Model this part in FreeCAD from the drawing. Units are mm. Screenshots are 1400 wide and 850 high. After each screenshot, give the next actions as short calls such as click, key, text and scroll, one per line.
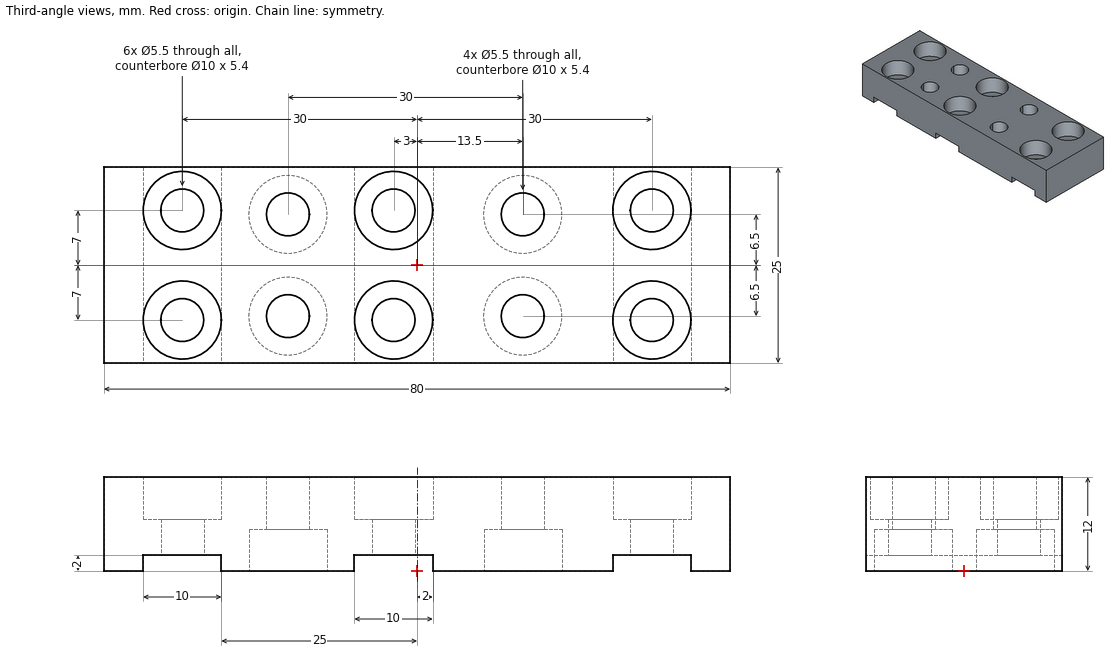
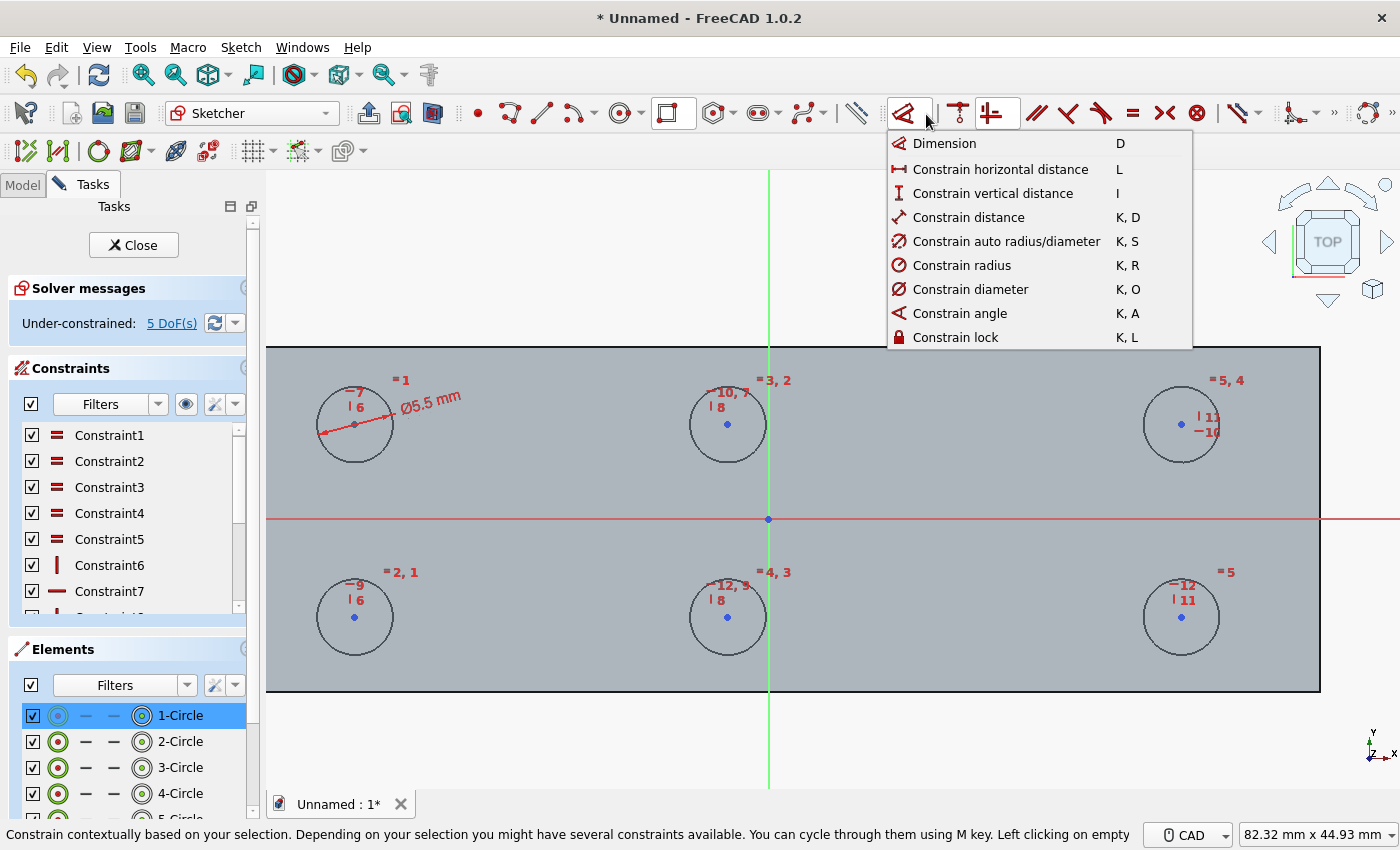
click(1040, 193)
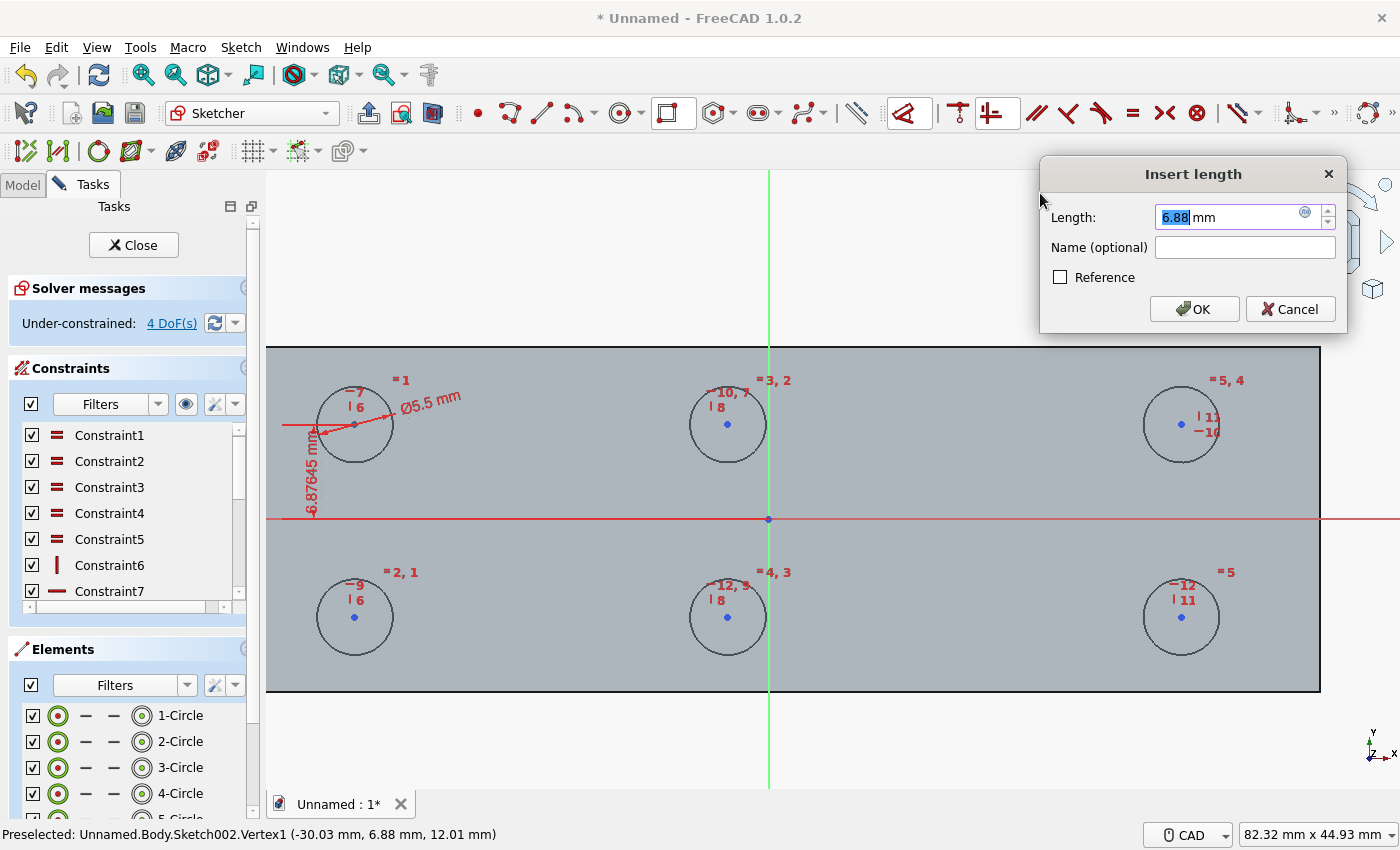
text(7)
key(Return)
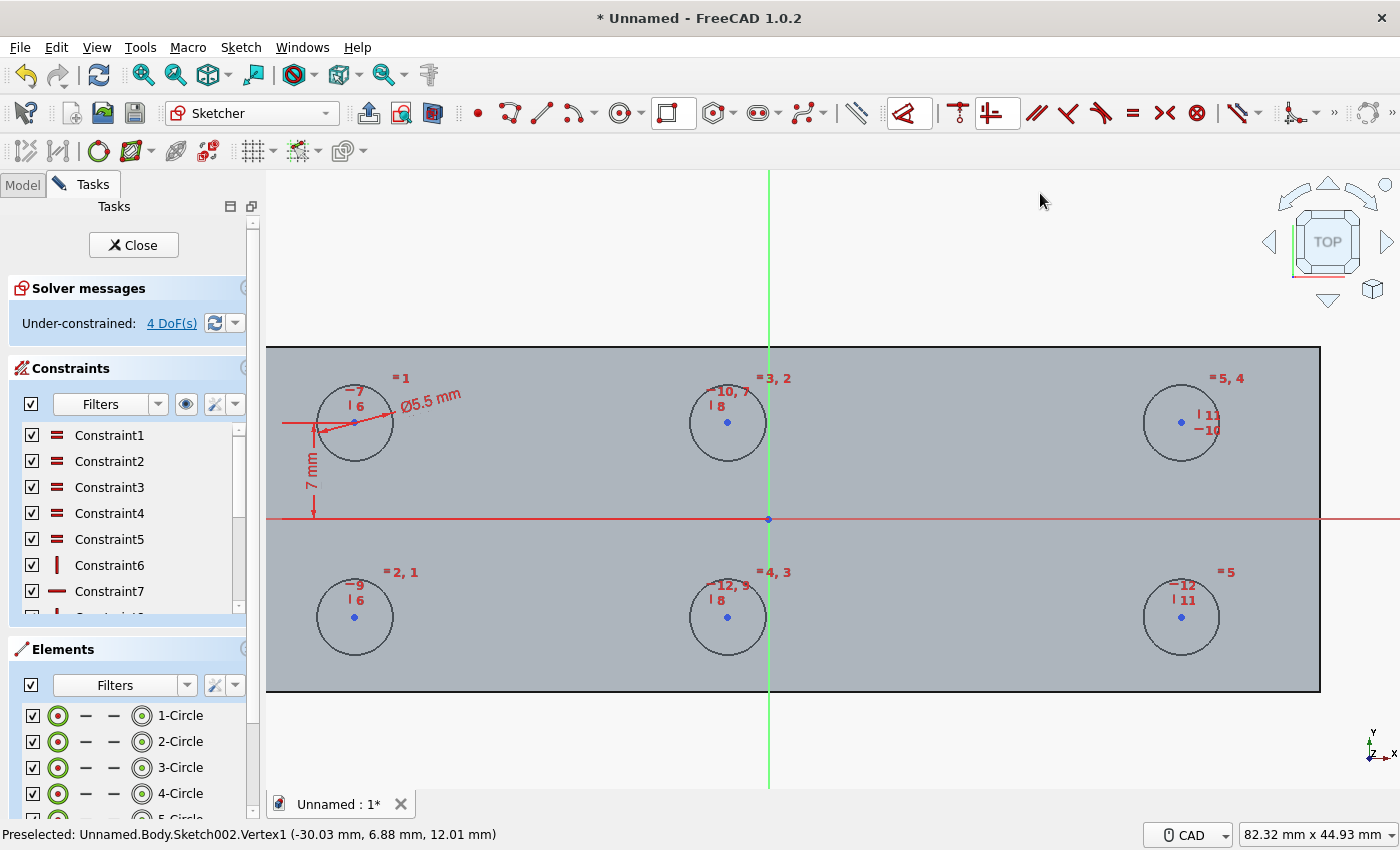
click(355, 617)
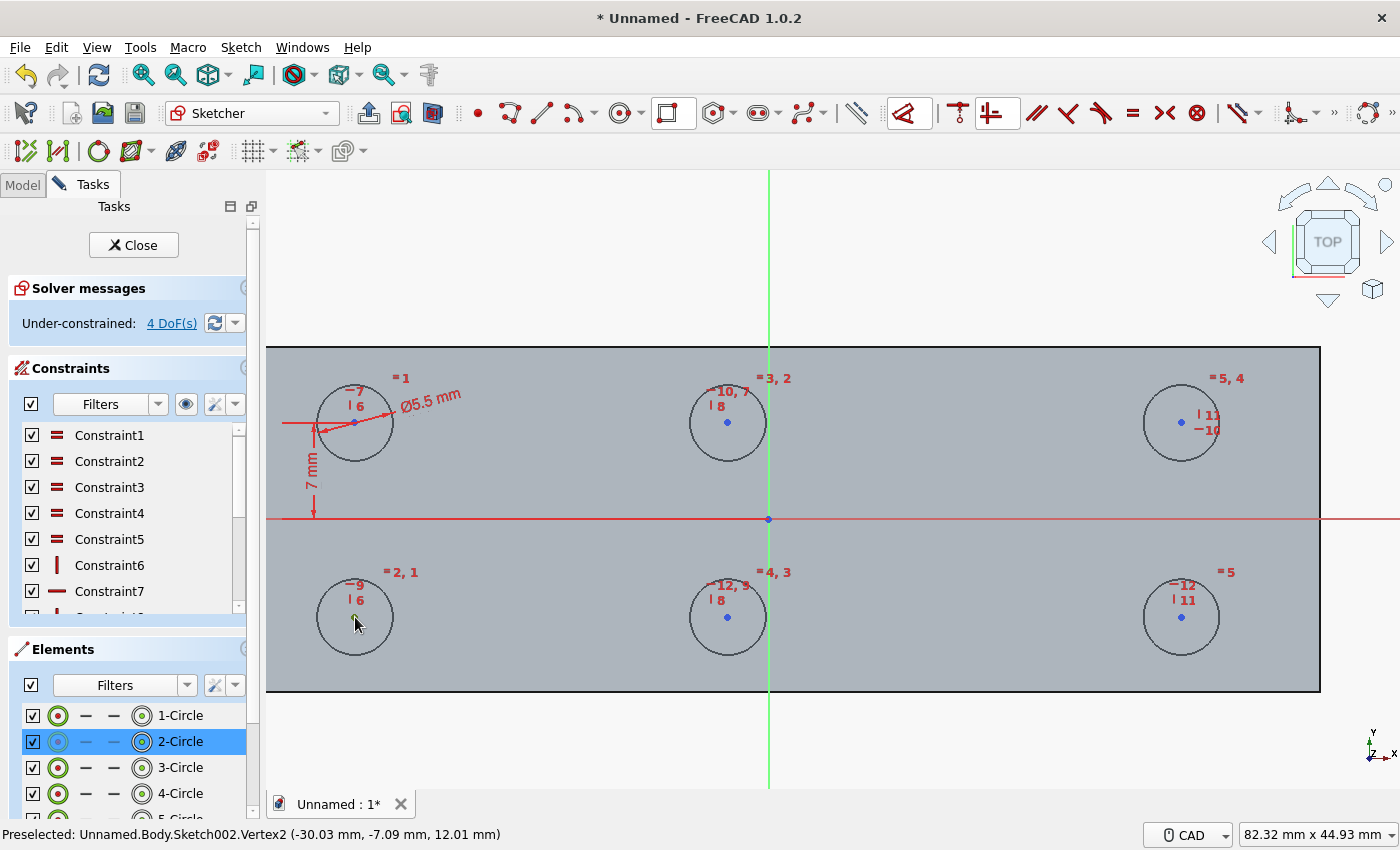
click(926, 114)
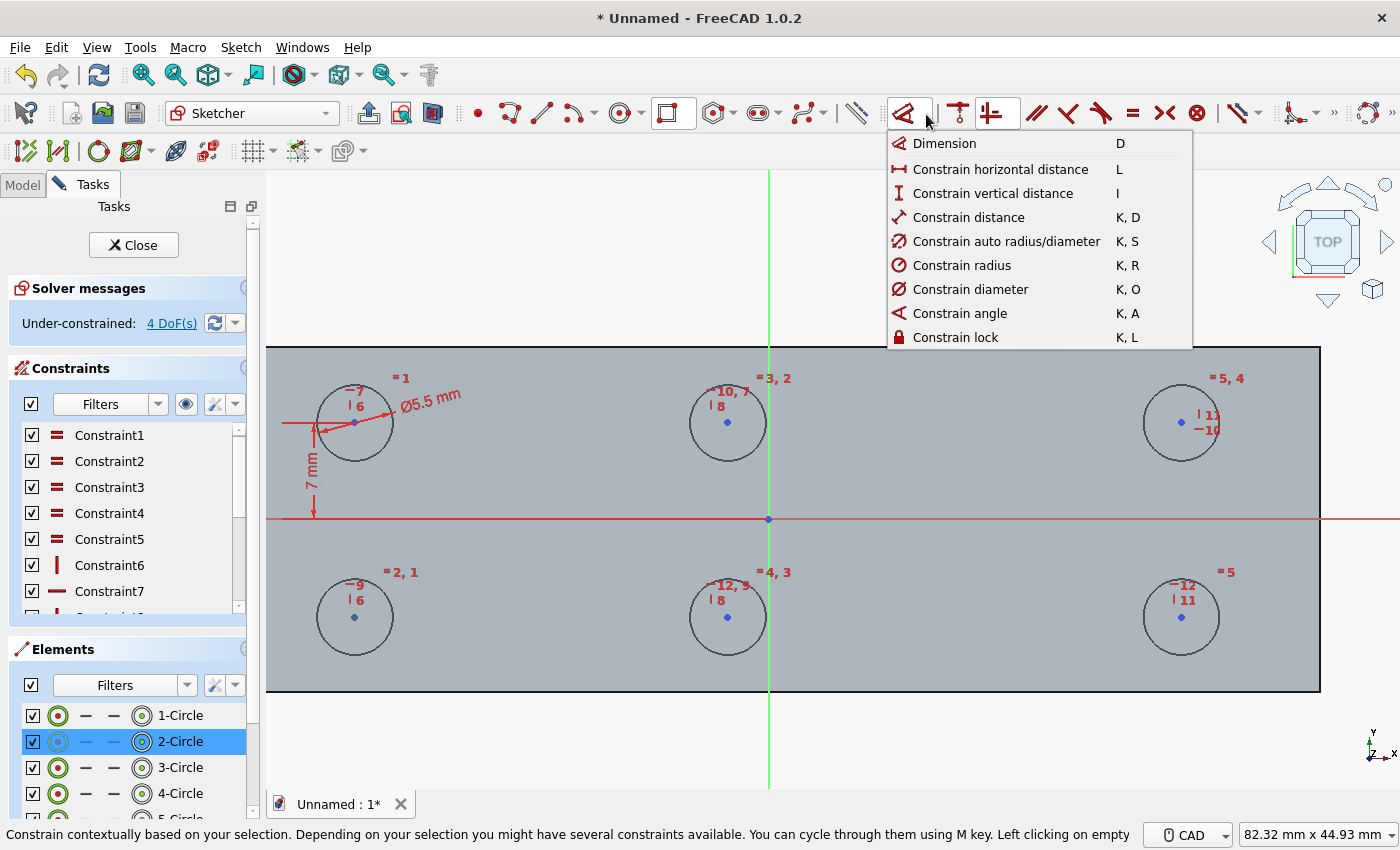
click(1040, 193)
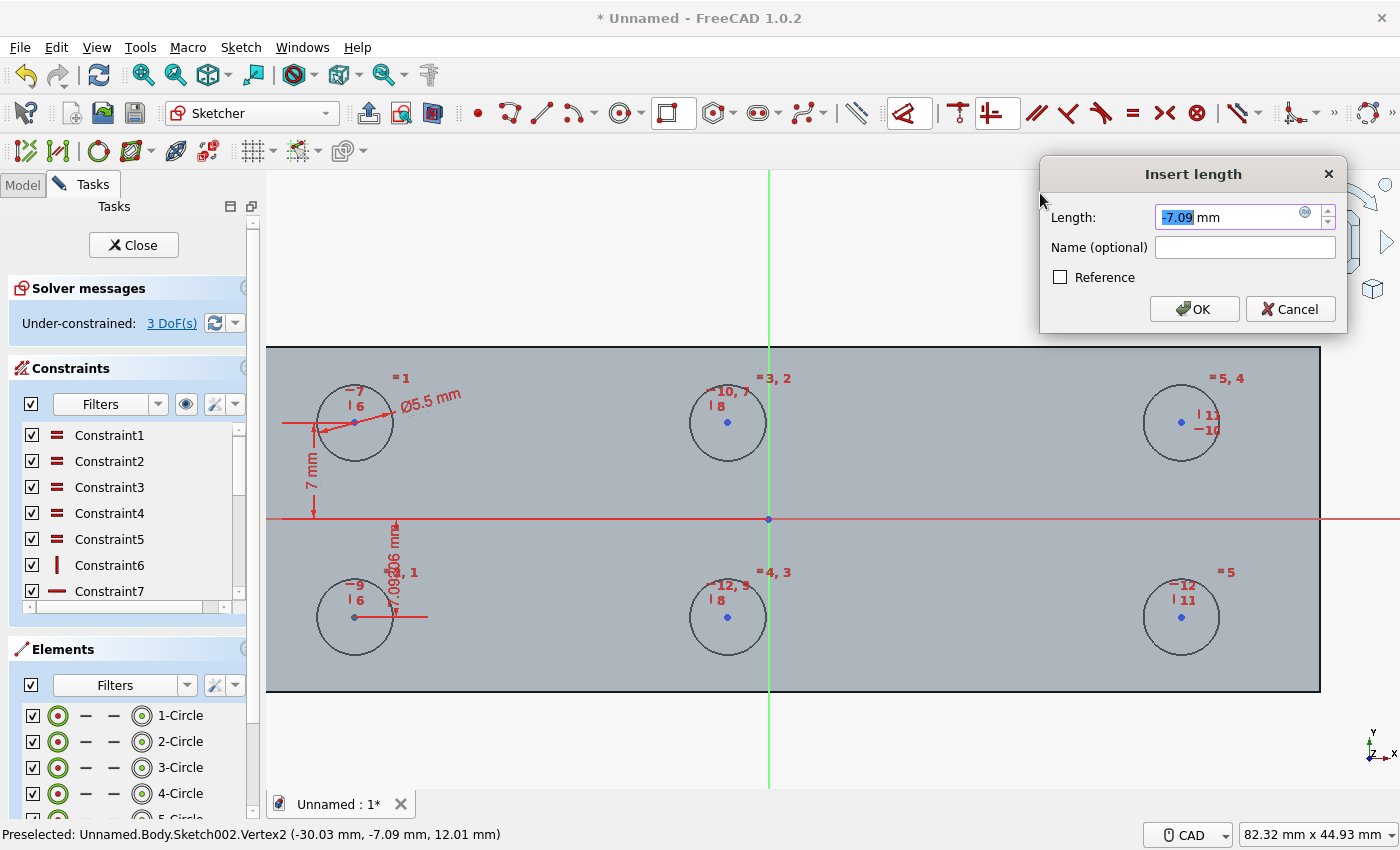
text(-7)
key(Return)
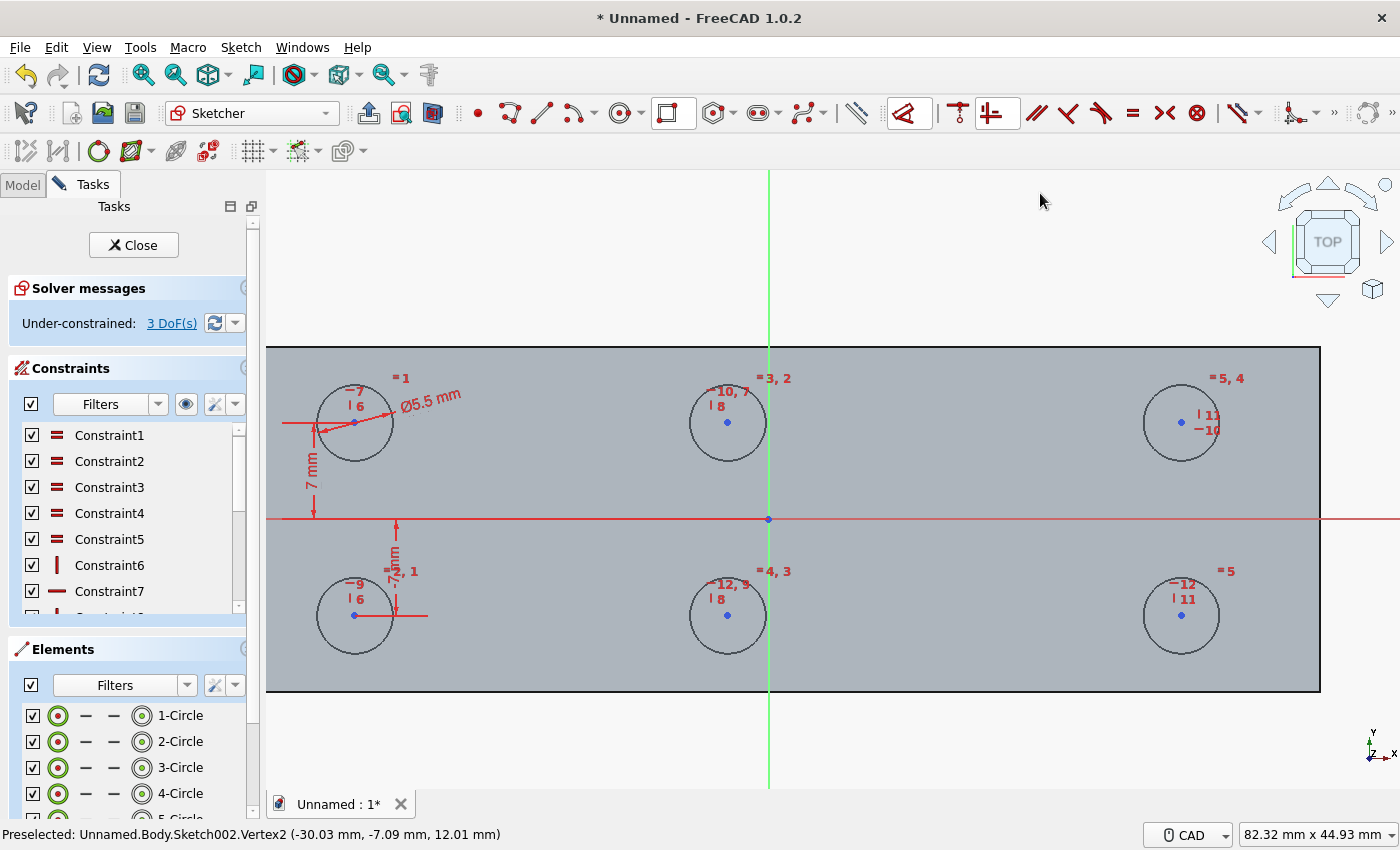
click(728, 423)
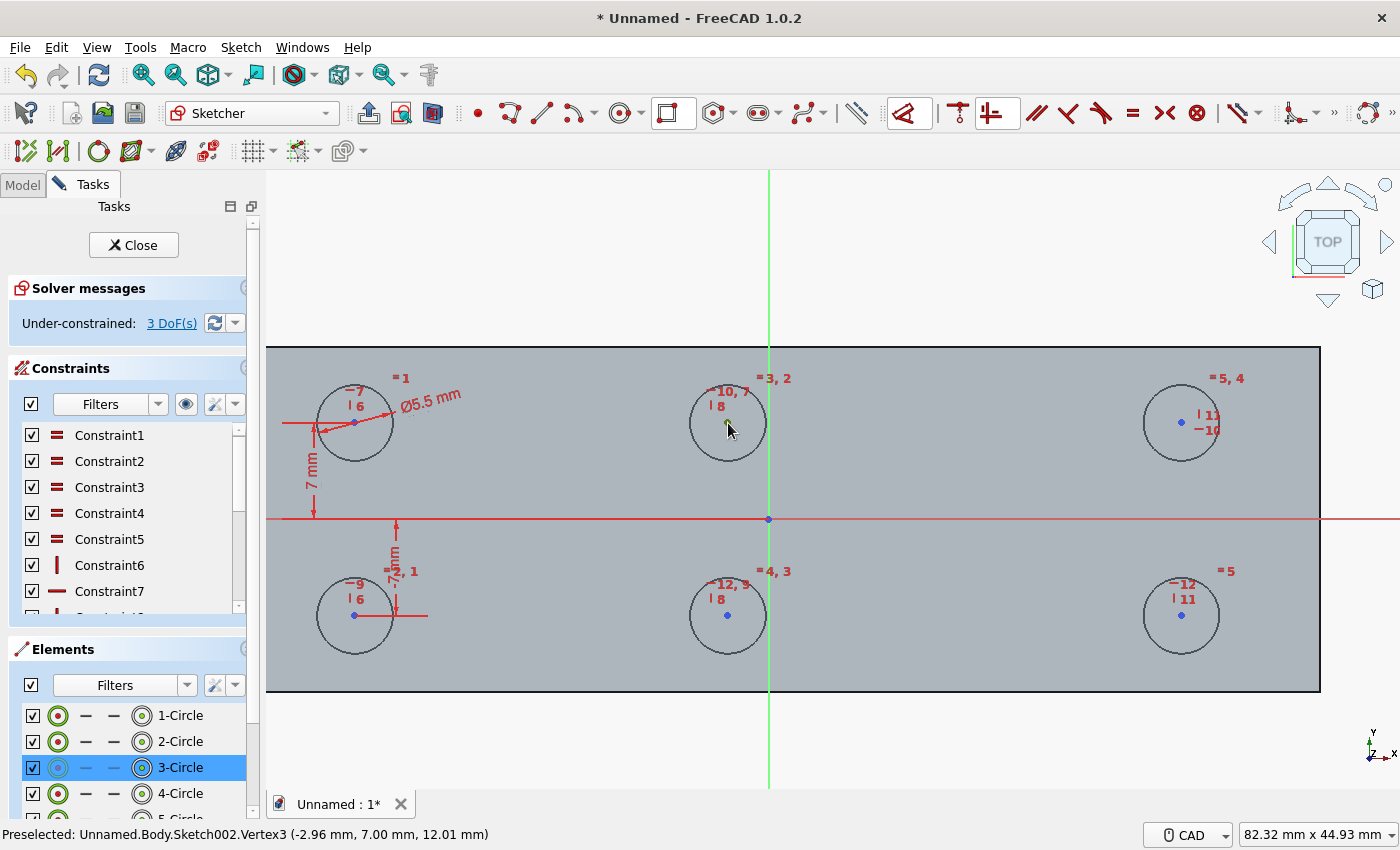
click(926, 114)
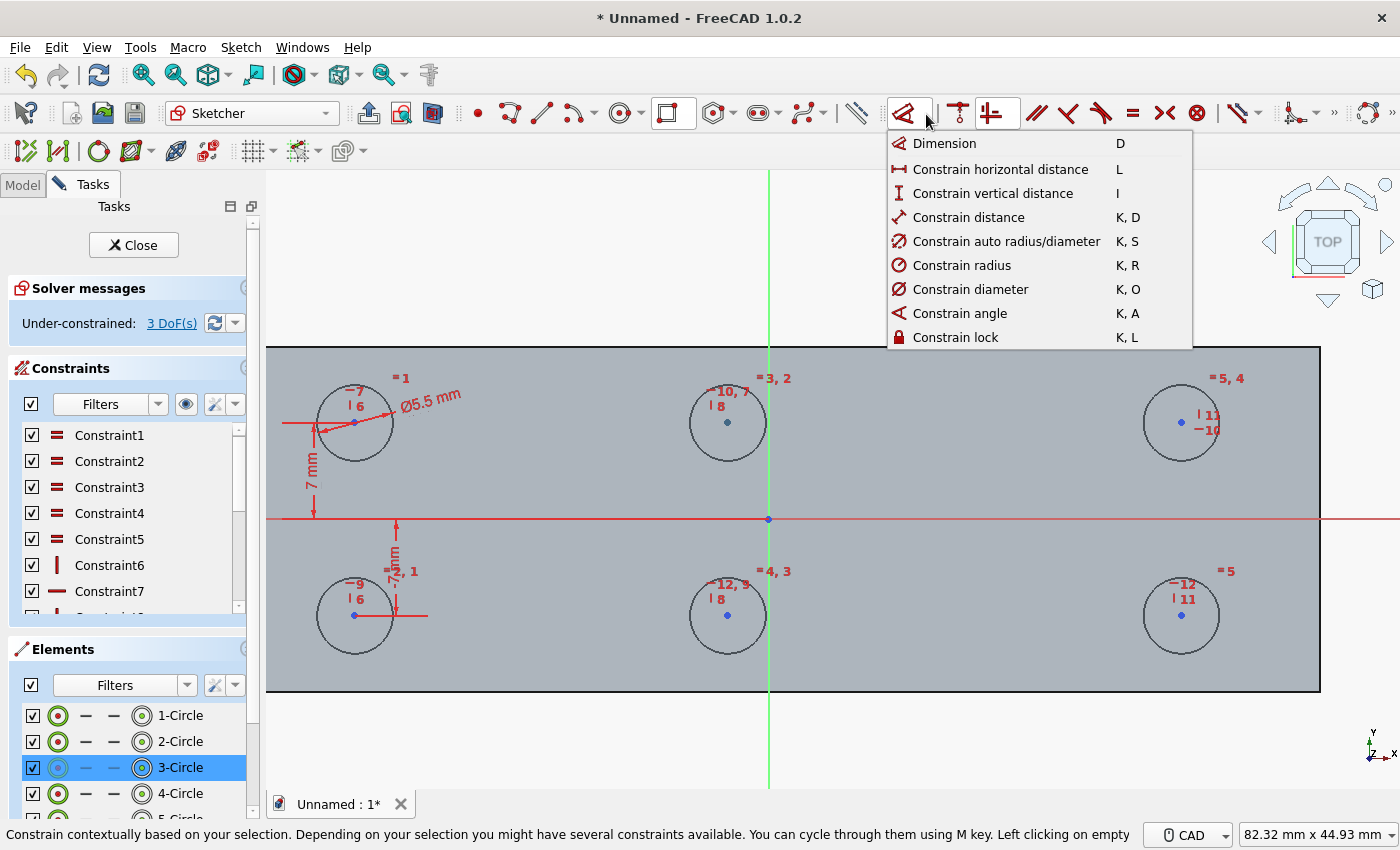
click(1040, 169)